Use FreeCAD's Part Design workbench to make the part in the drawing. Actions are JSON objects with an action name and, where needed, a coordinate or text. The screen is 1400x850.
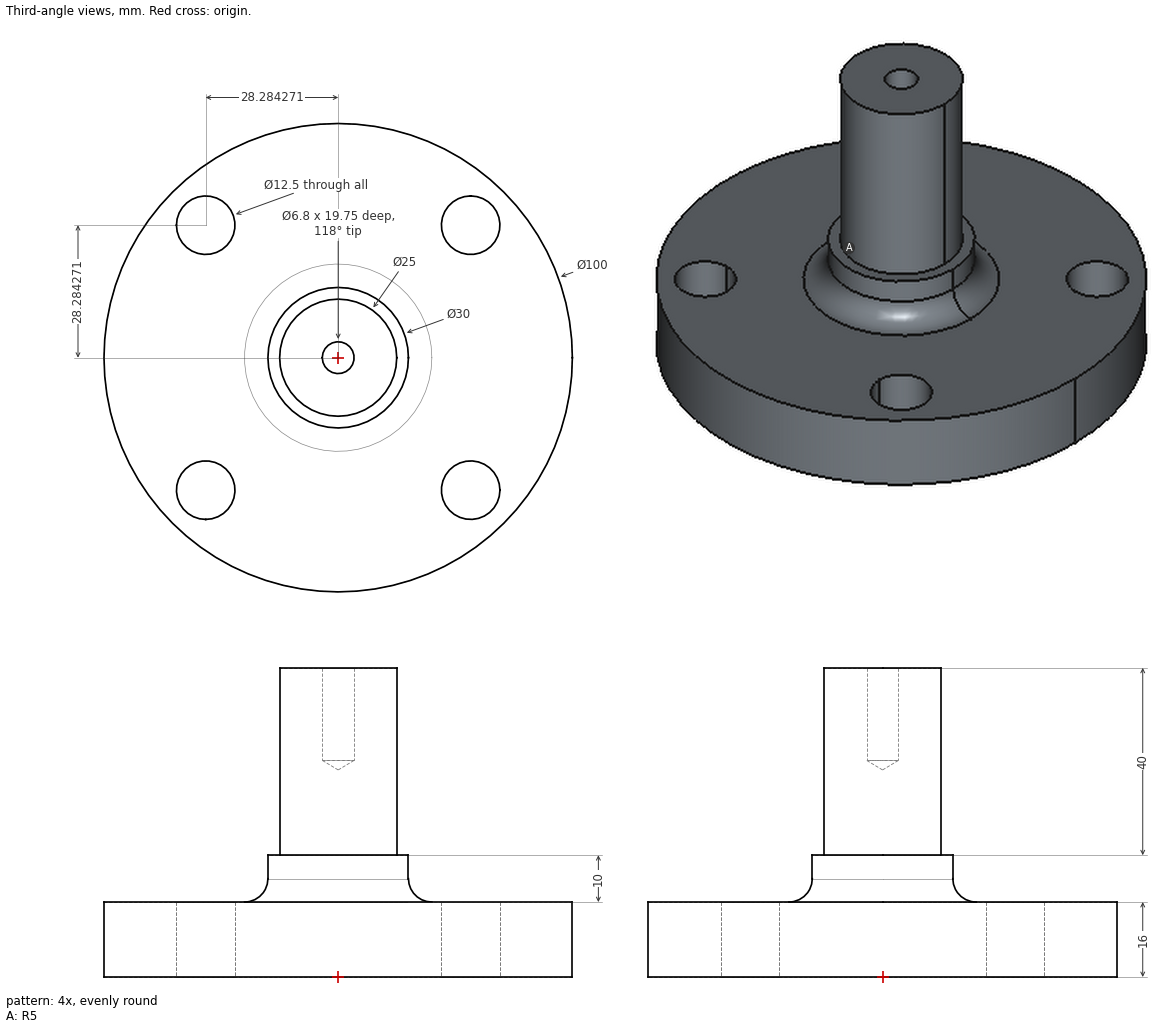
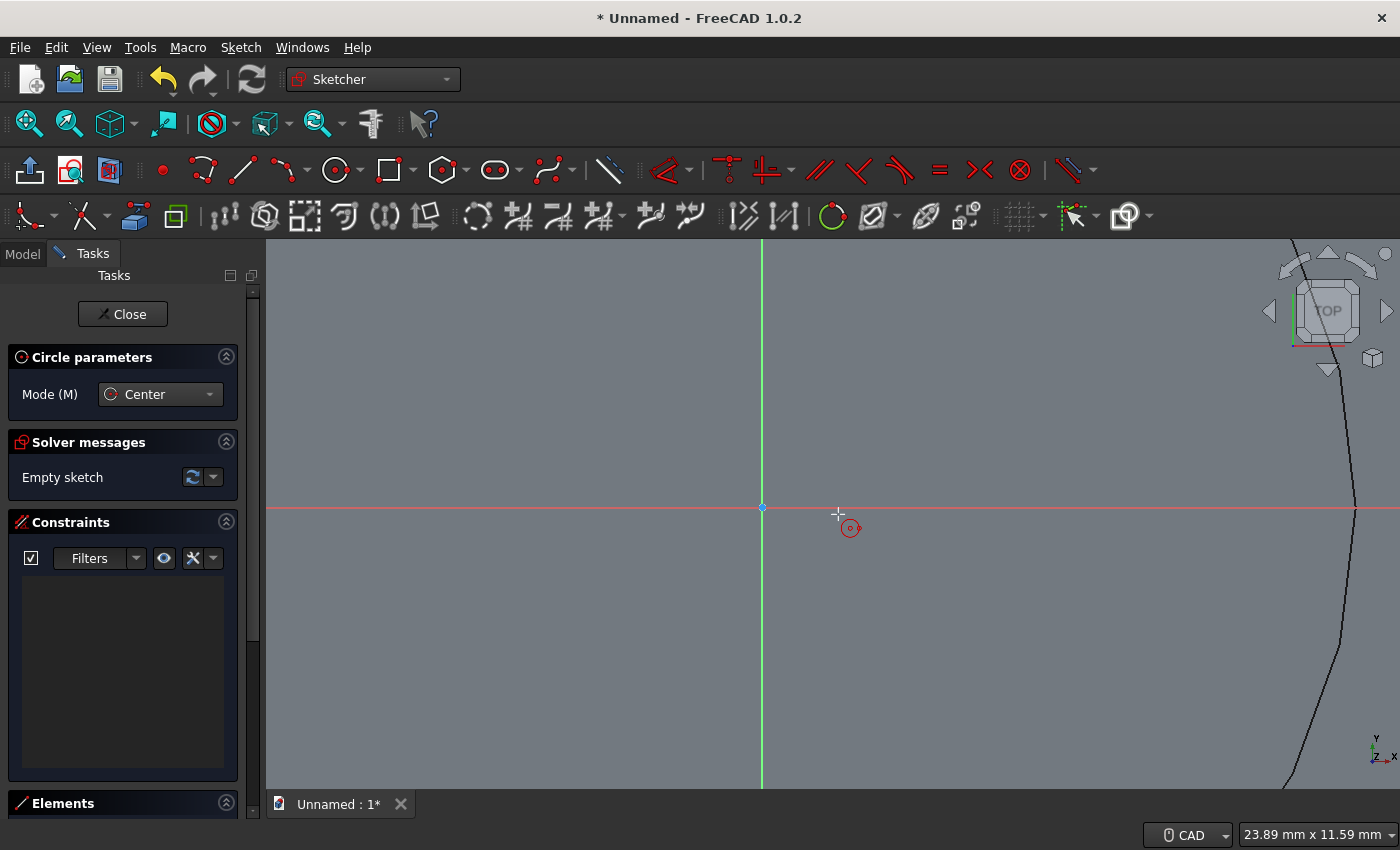
{"action": "left_click", "coordinate": [762, 508]}
{"action": "left_click", "coordinate": [876, 394]}
{"action": "key", "text": "Escape"}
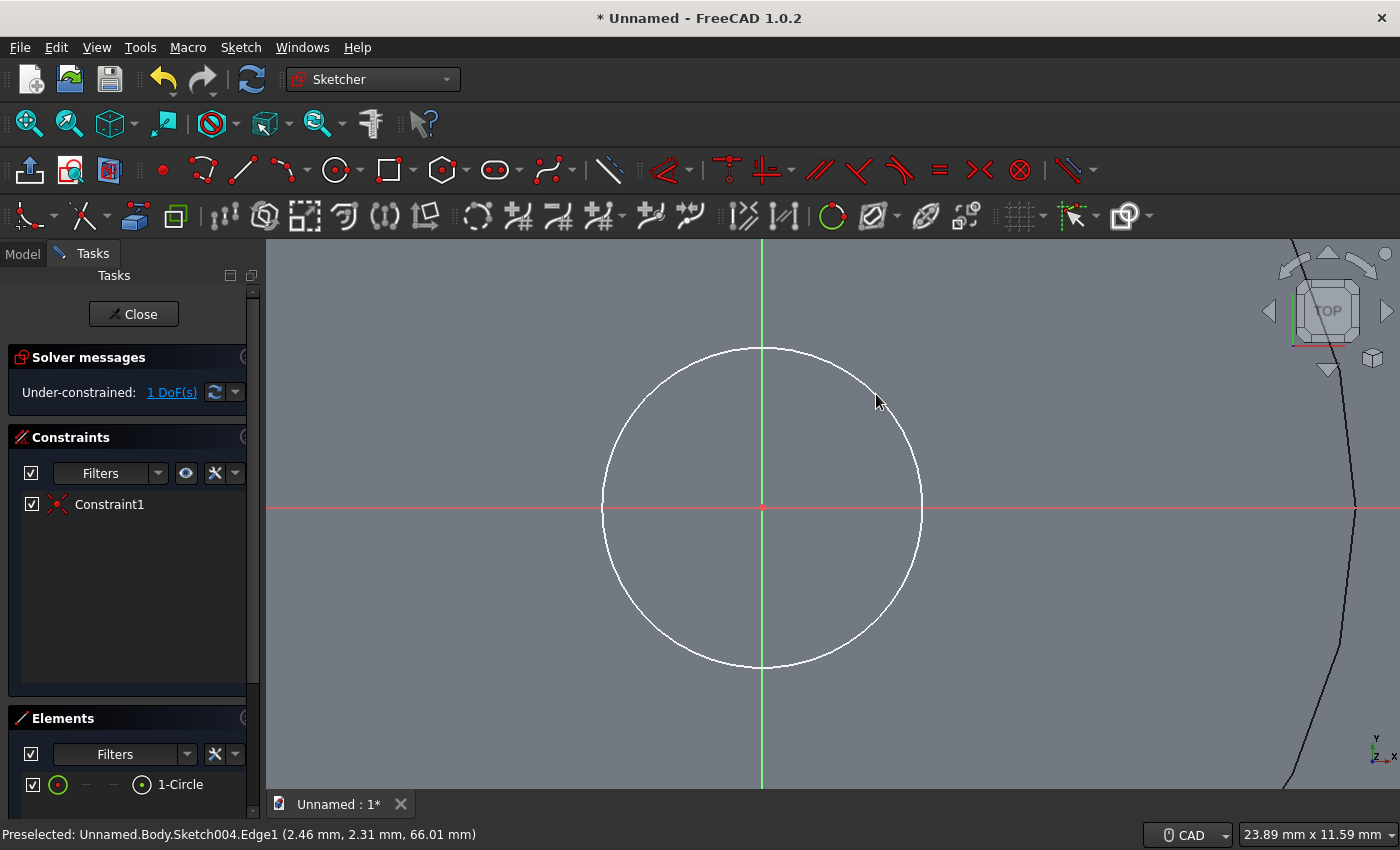
{"action": "left_click", "coordinate": [664, 170]}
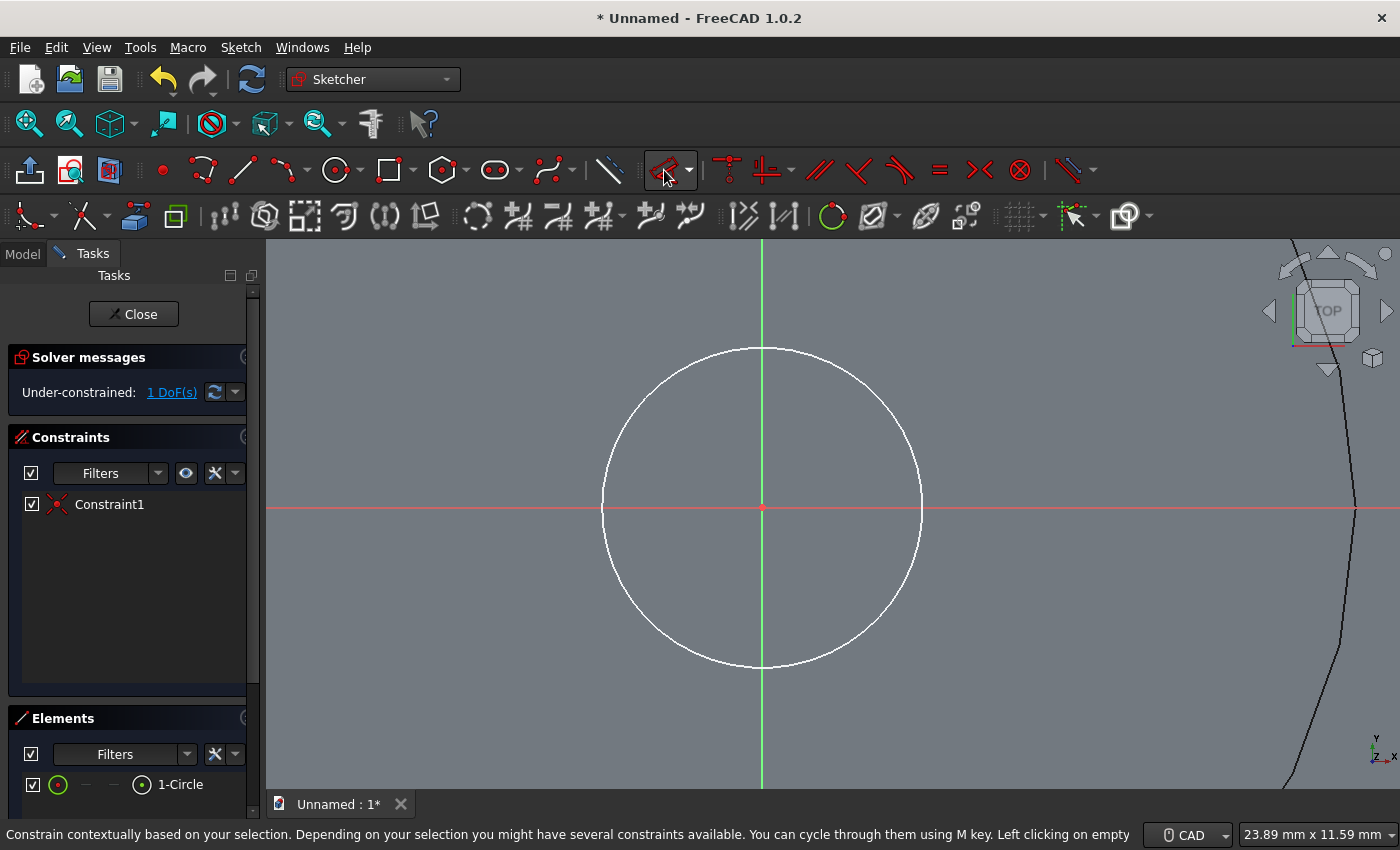
{"action": "left_click", "coordinate": [875, 394]}
{"action": "left_click", "coordinate": [898, 371]}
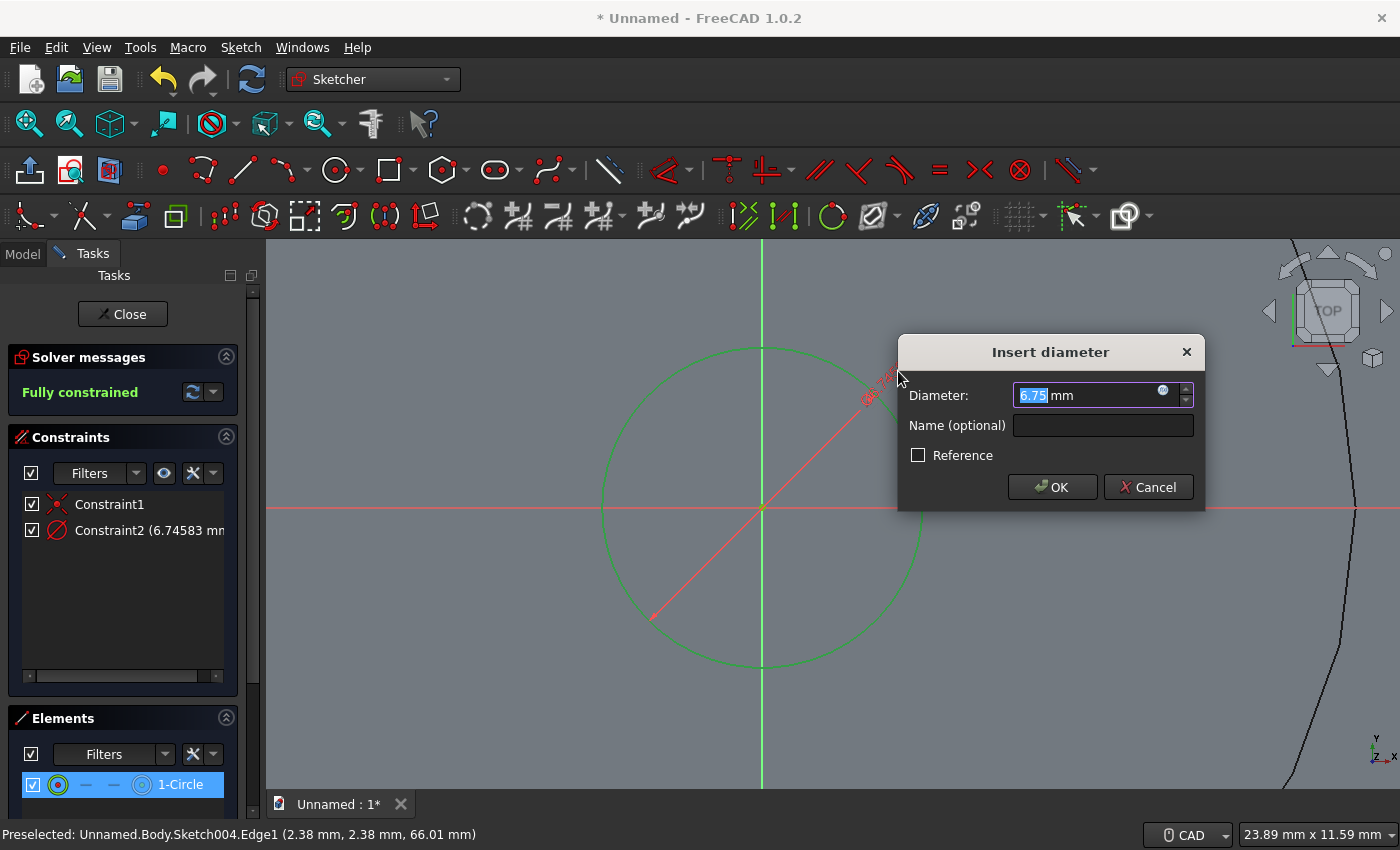
{"action": "type", "text": "6.8"}
{"action": "key", "text": "Return"}
{"action": "key", "text": "Escape"}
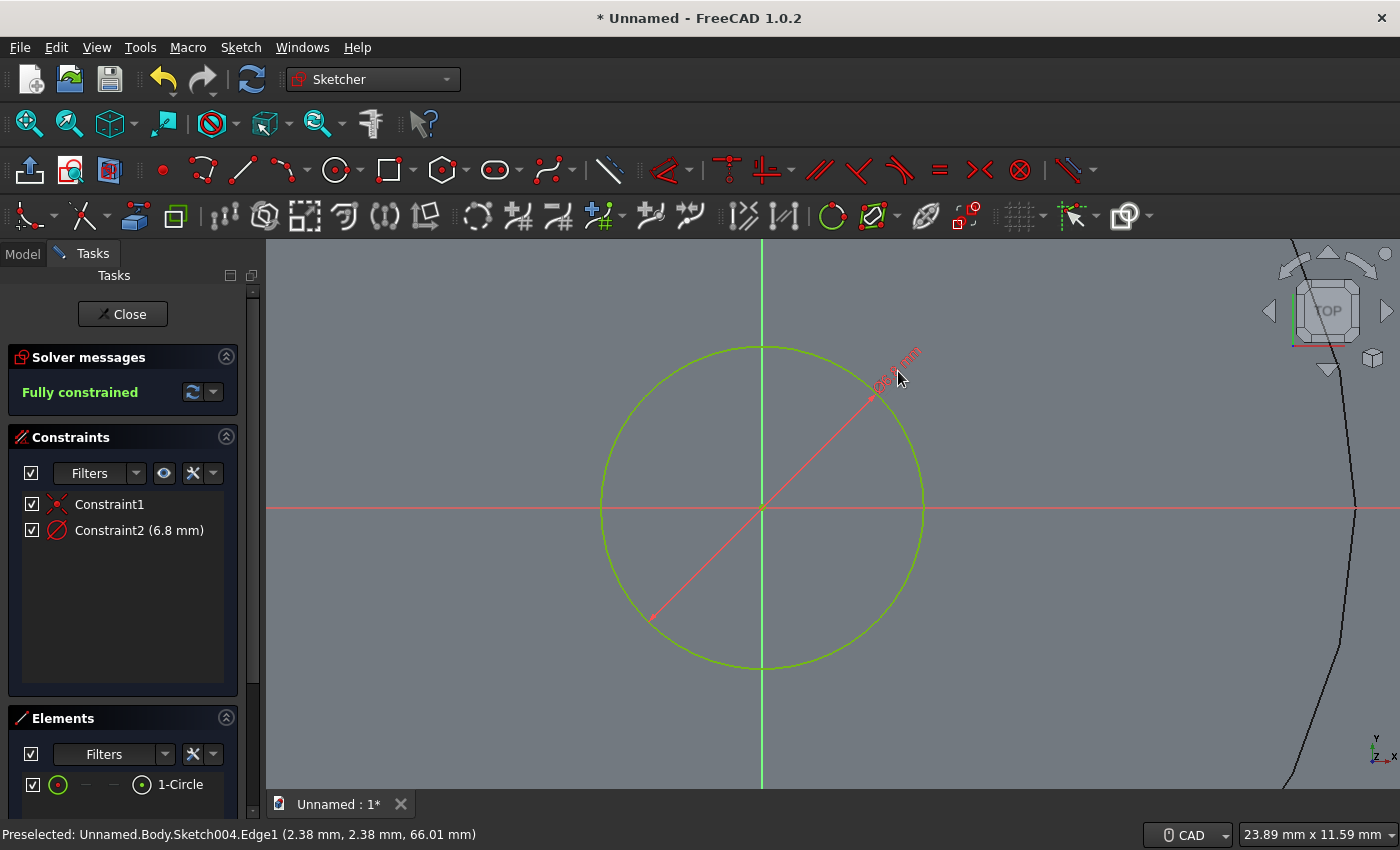
{"action": "left_click", "coordinate": [123, 314]}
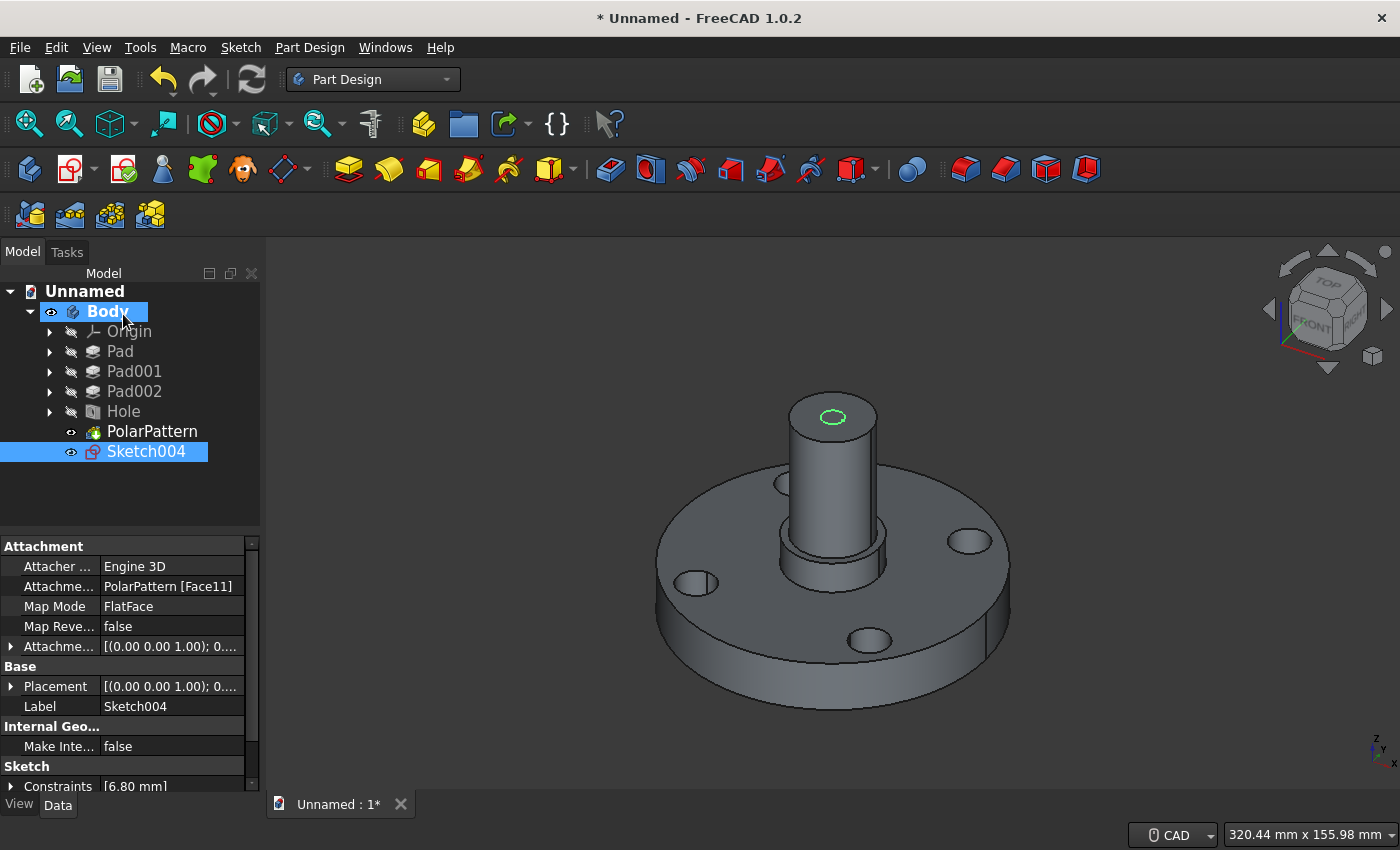
{"action": "left_click", "coordinate": [652, 170]}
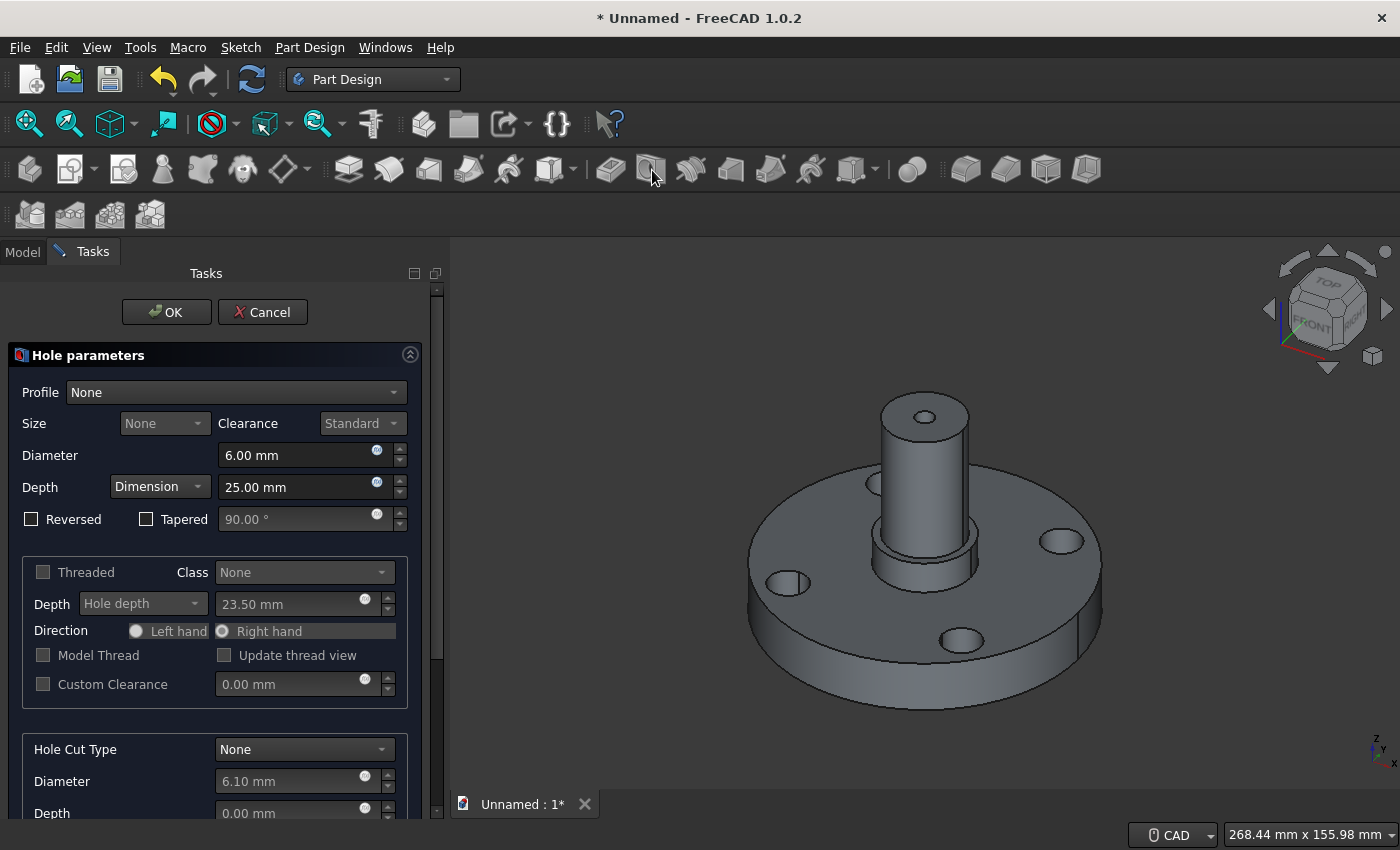
{"action": "triple_click", "coordinate": [305, 455]}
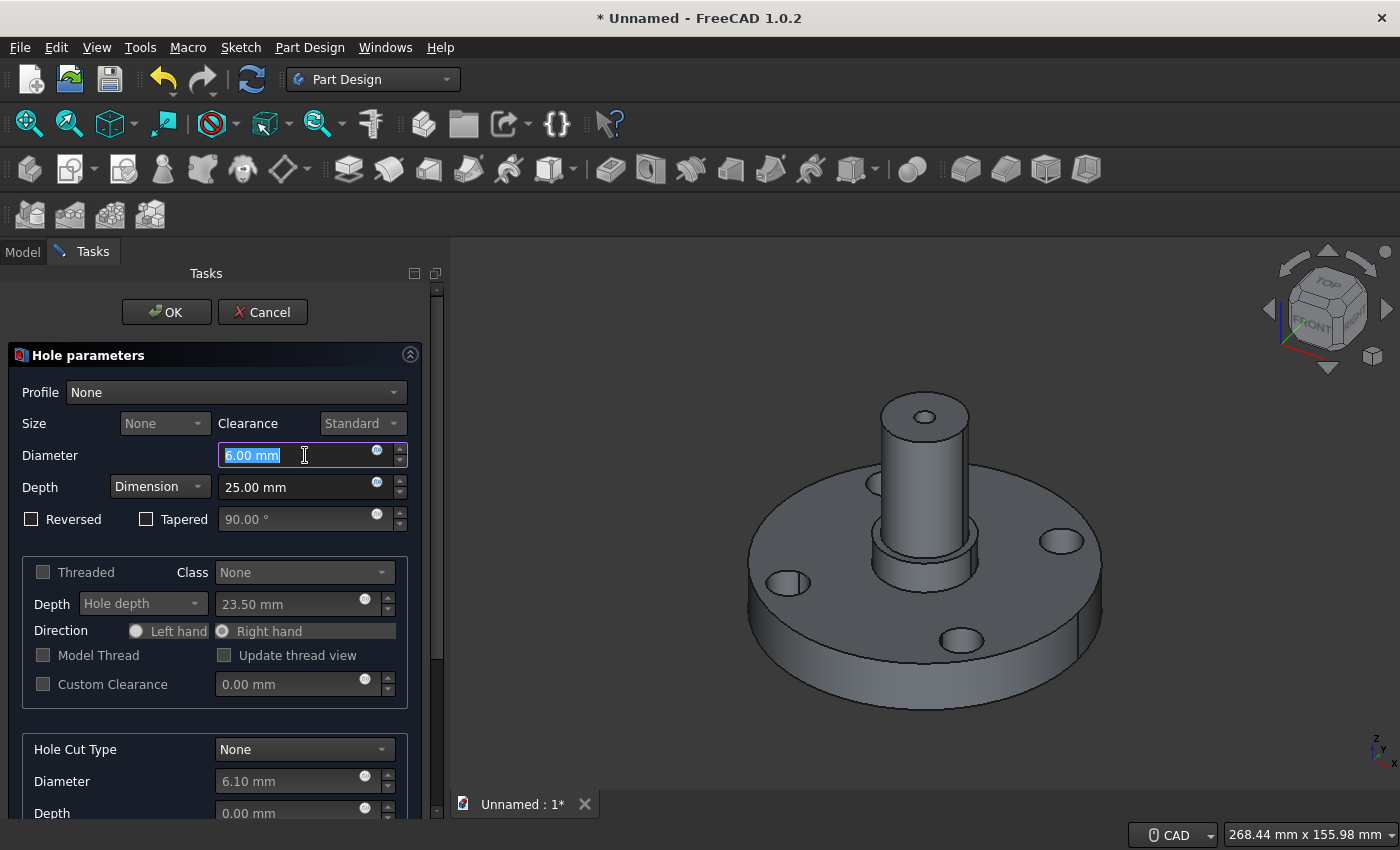
{"action": "type", "text": "6.8"}
{"action": "key", "text": "Tab"}